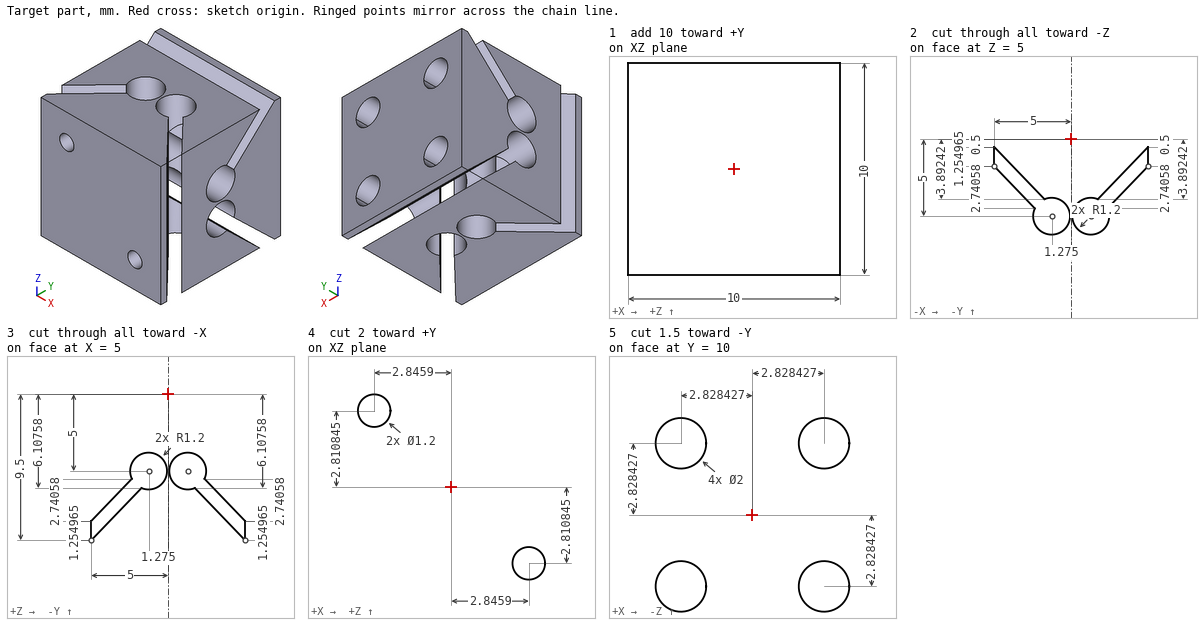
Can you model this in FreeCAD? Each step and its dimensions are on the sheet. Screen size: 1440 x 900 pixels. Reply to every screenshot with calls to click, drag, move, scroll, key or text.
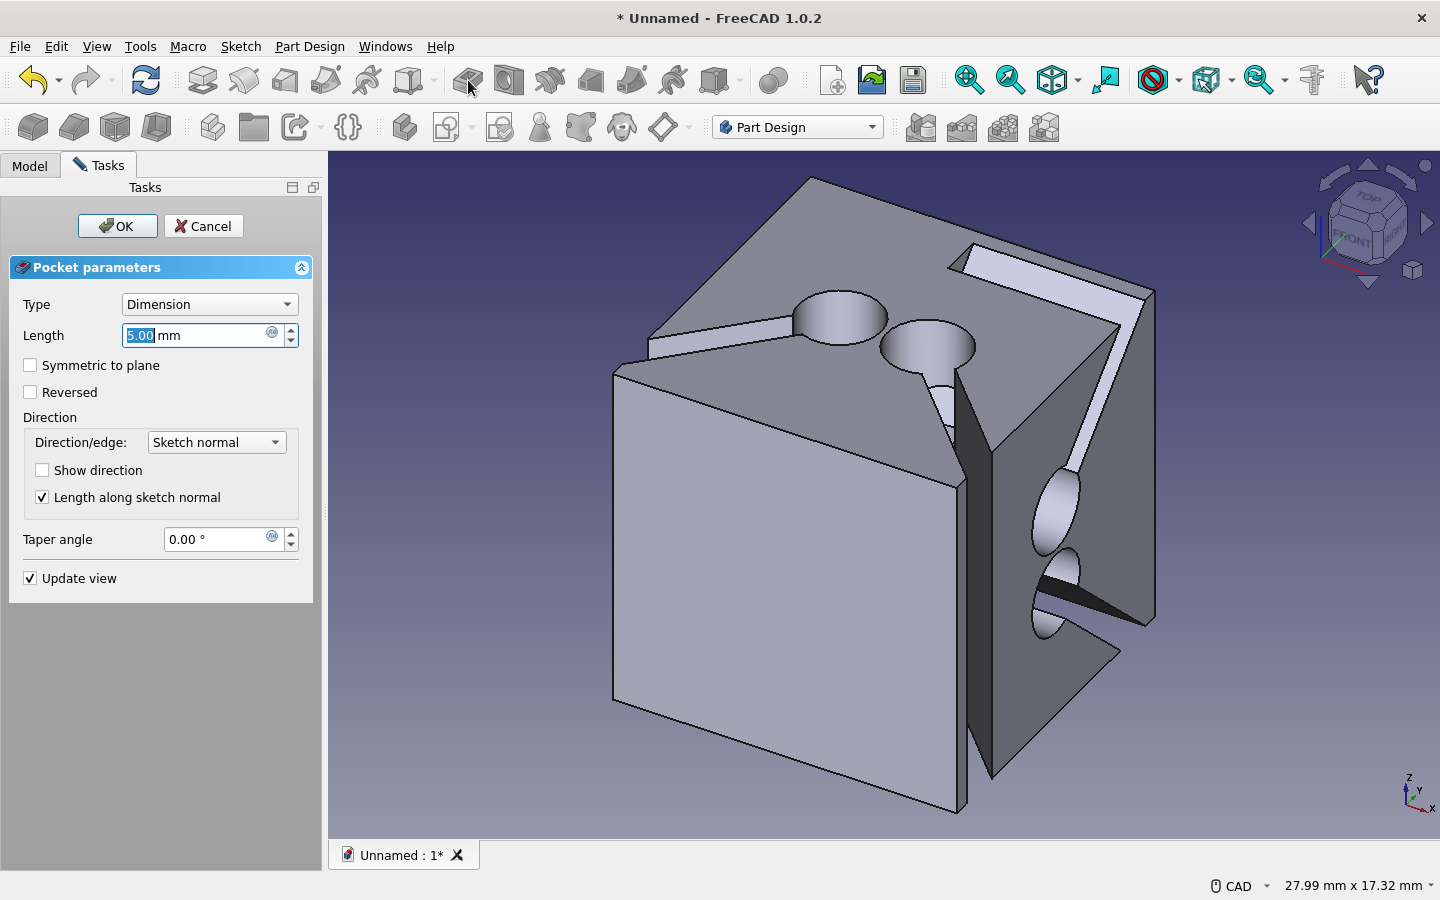
click(210, 304)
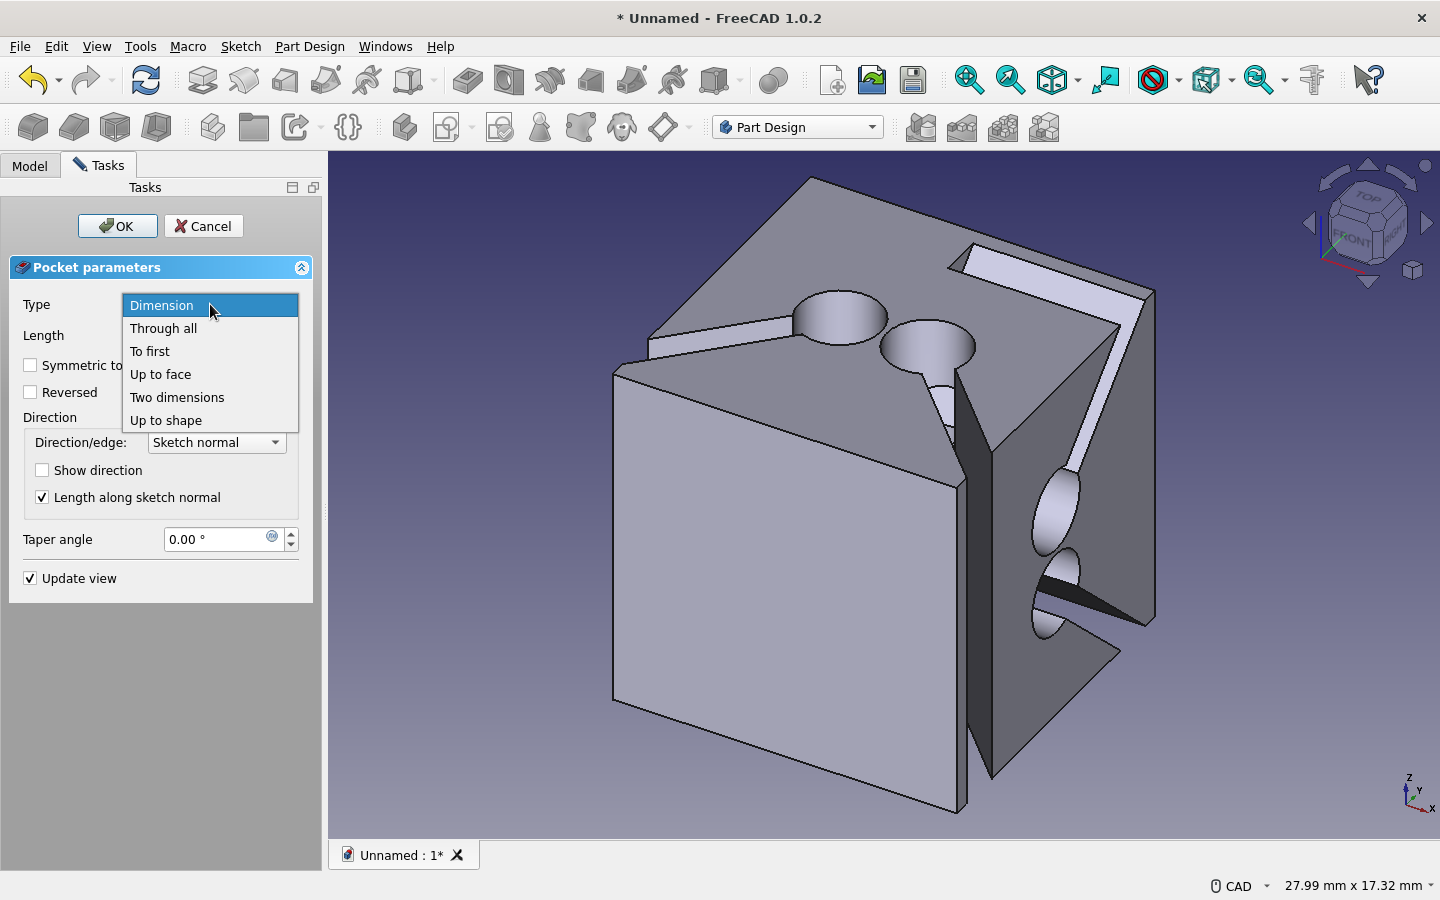
click(208, 328)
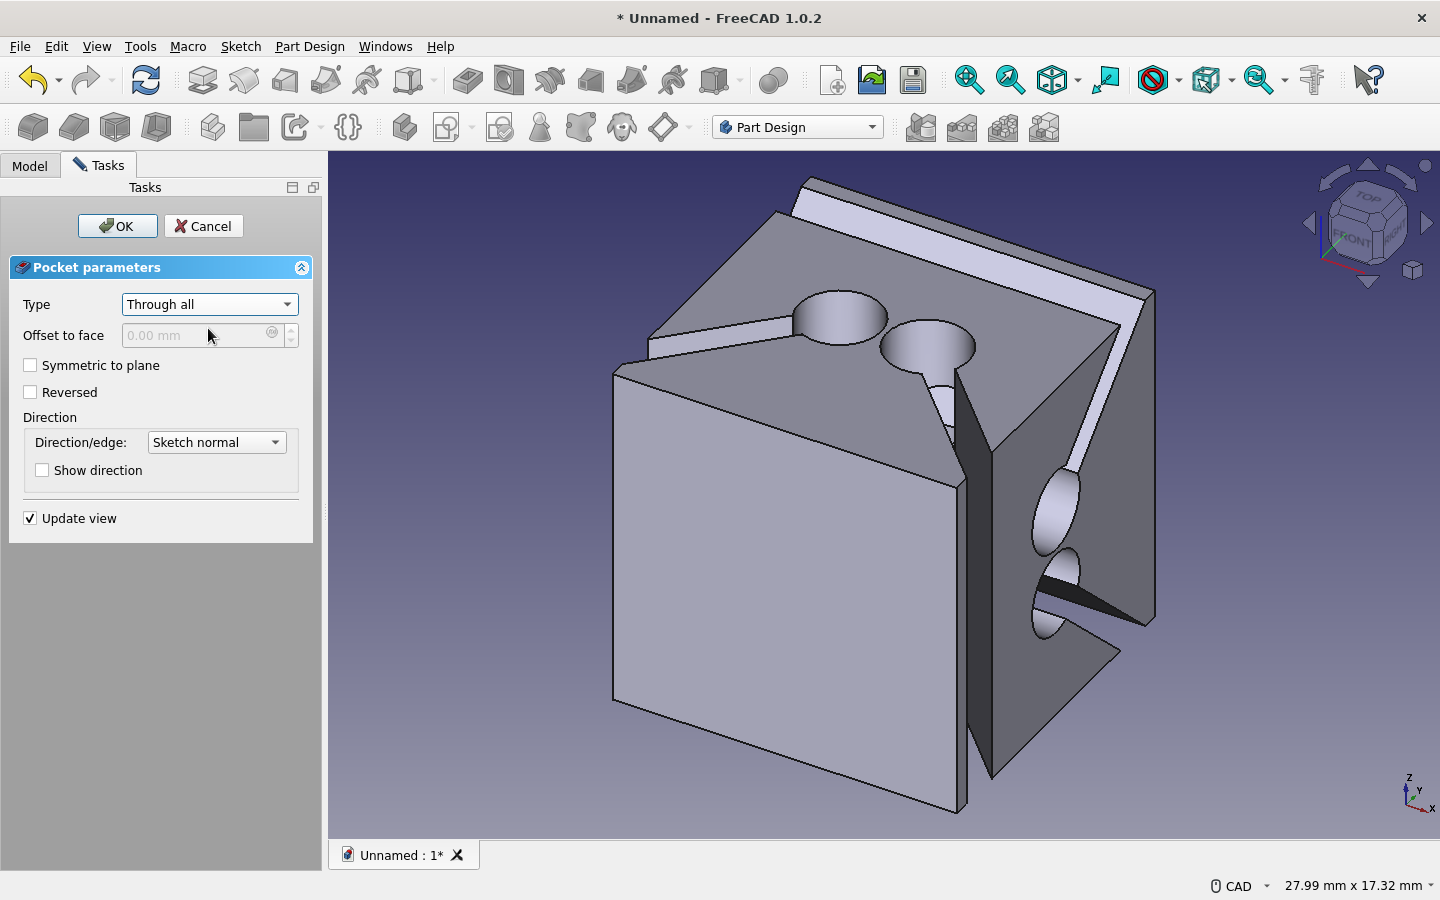
click(118, 226)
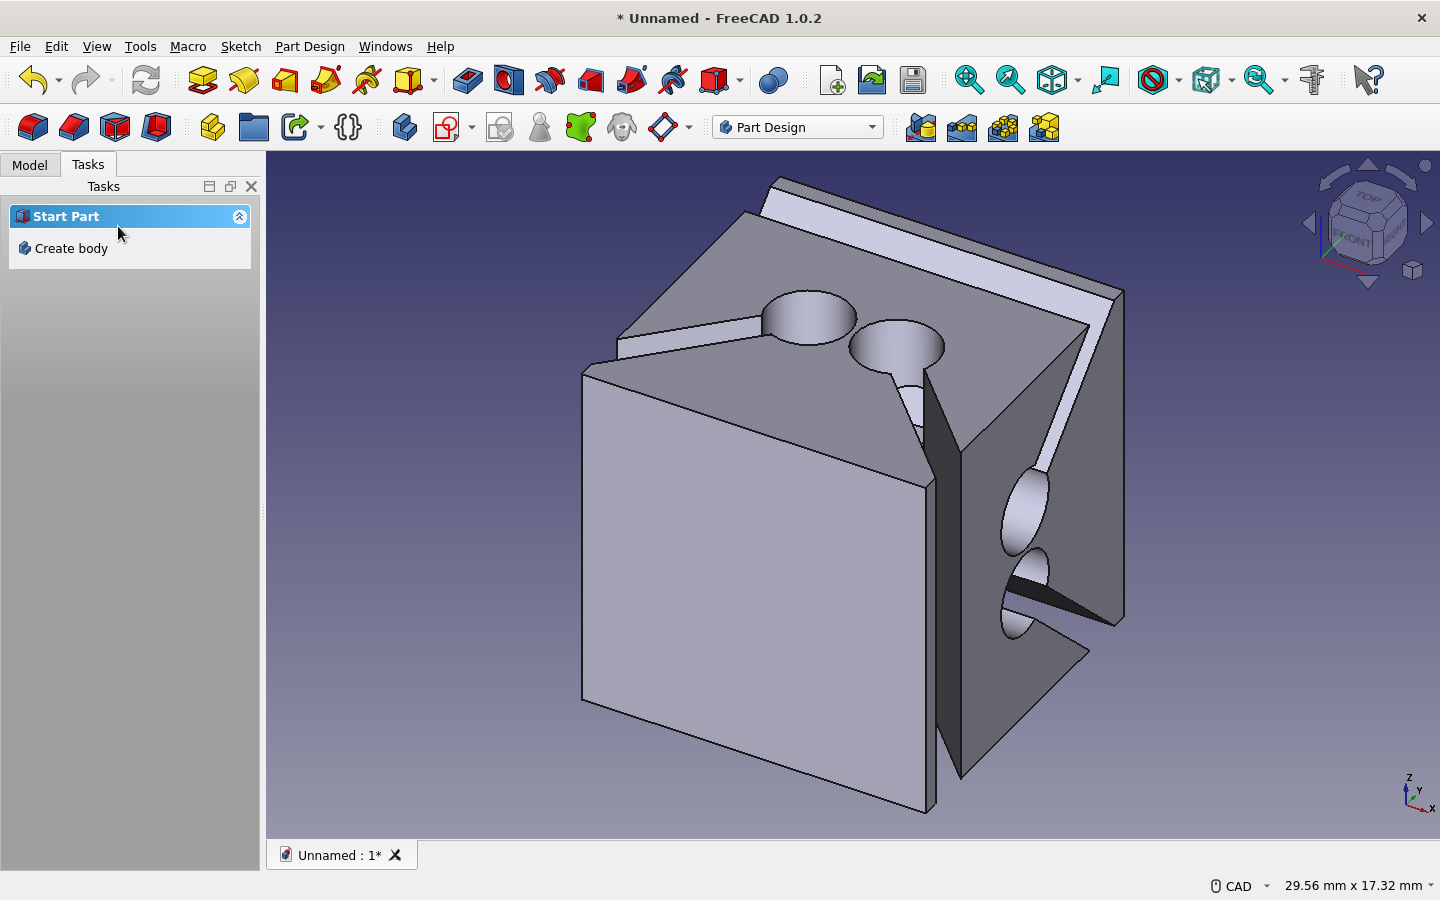
click(446, 128)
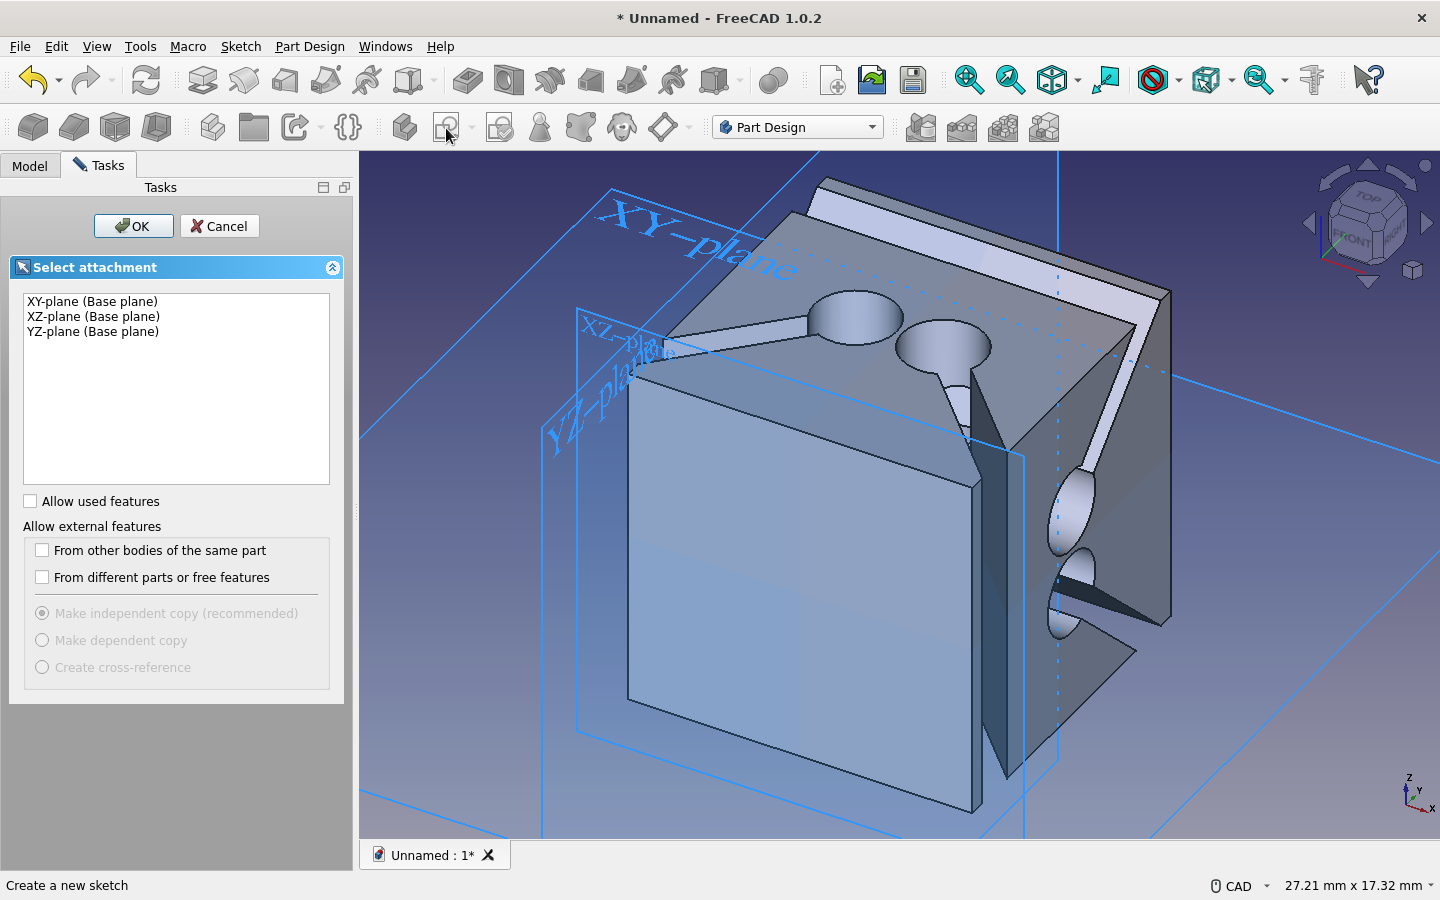
click(84, 316)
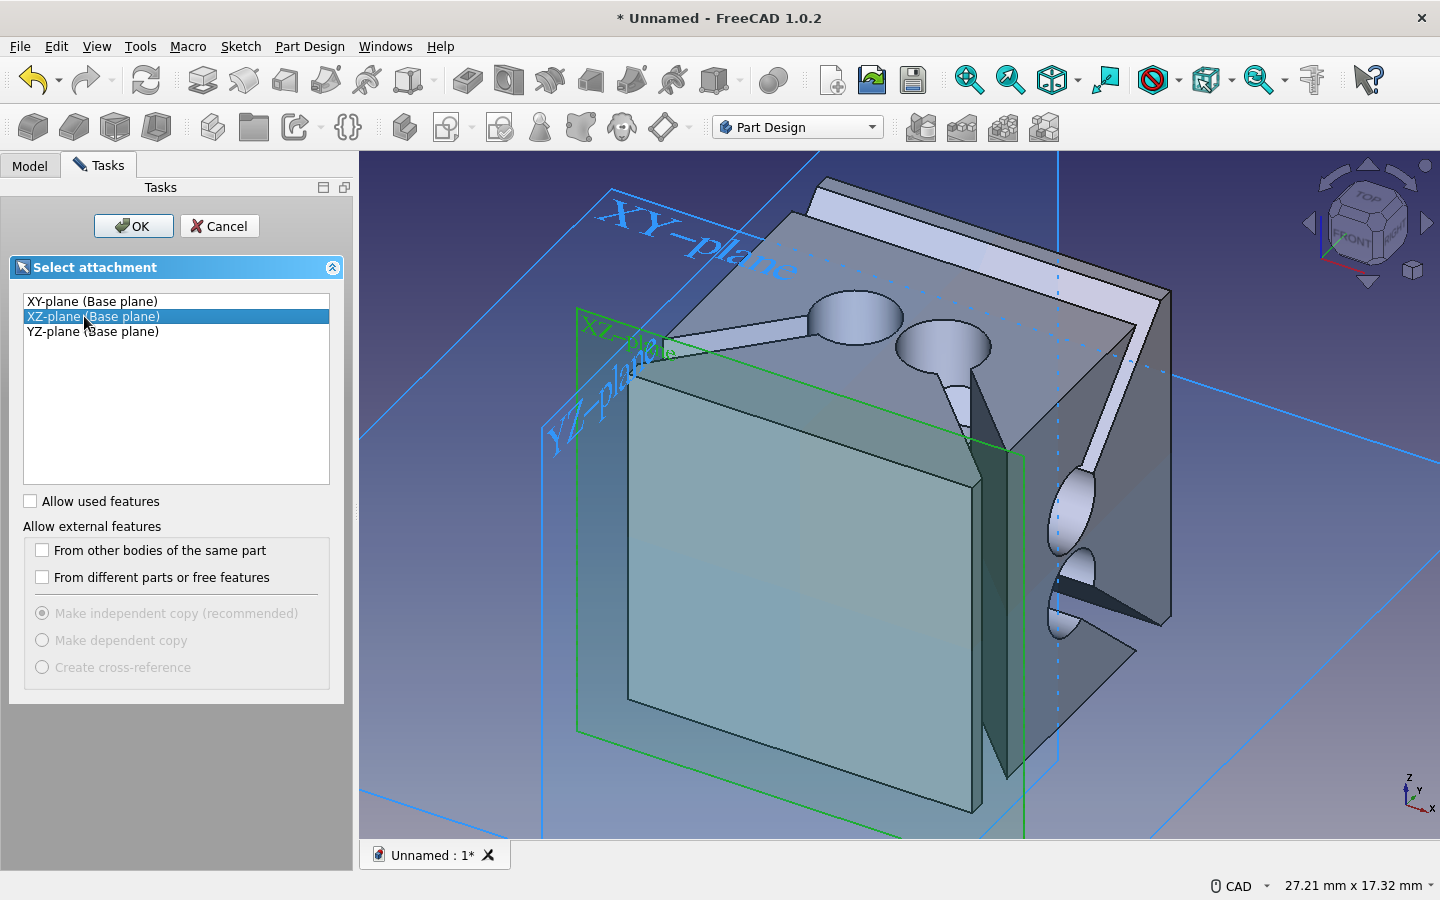
click(134, 226)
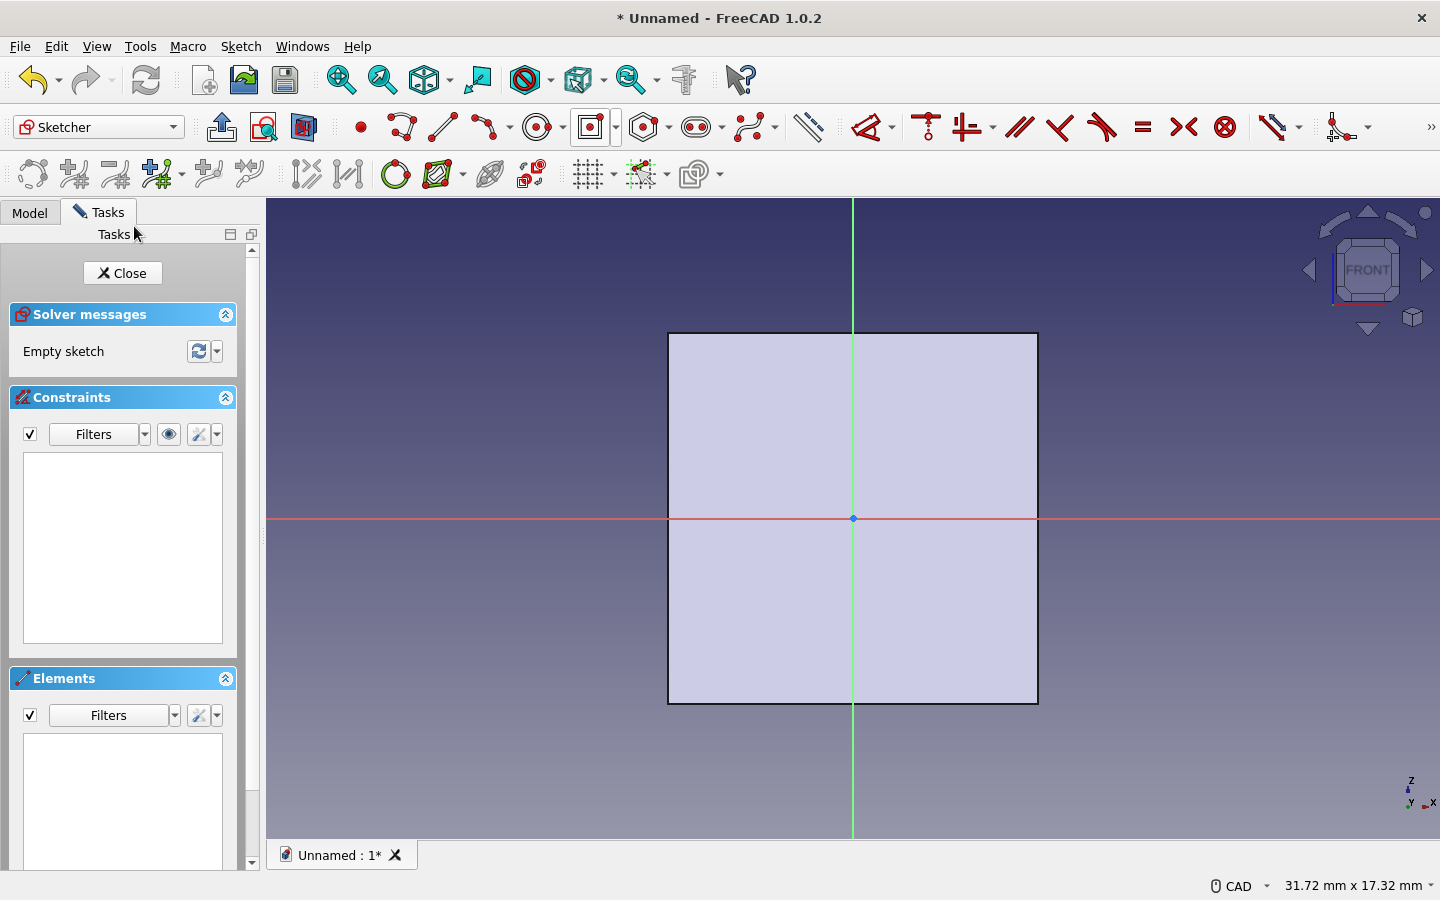
scroll(992, 519, up, 2)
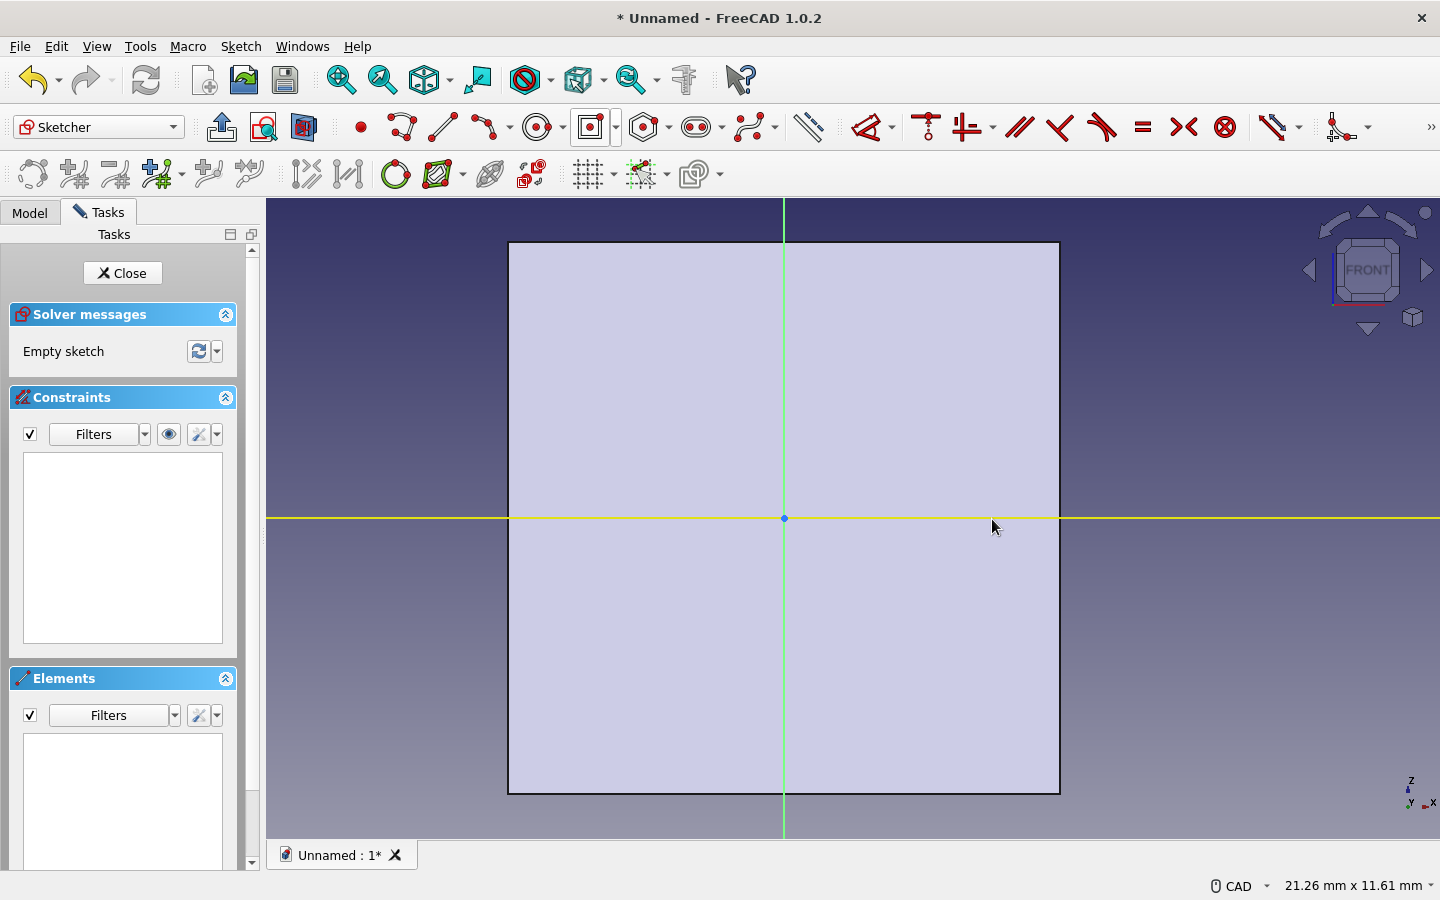
click(536, 128)